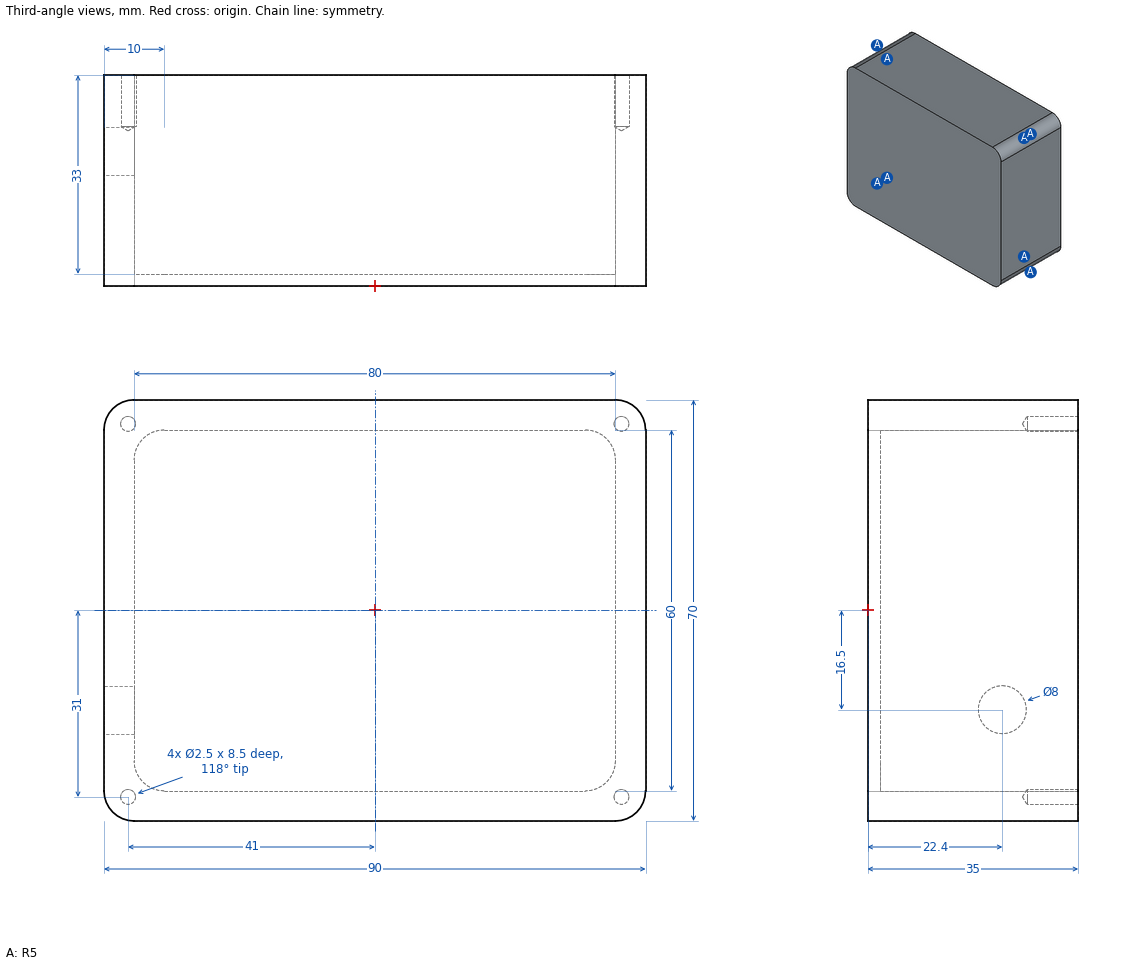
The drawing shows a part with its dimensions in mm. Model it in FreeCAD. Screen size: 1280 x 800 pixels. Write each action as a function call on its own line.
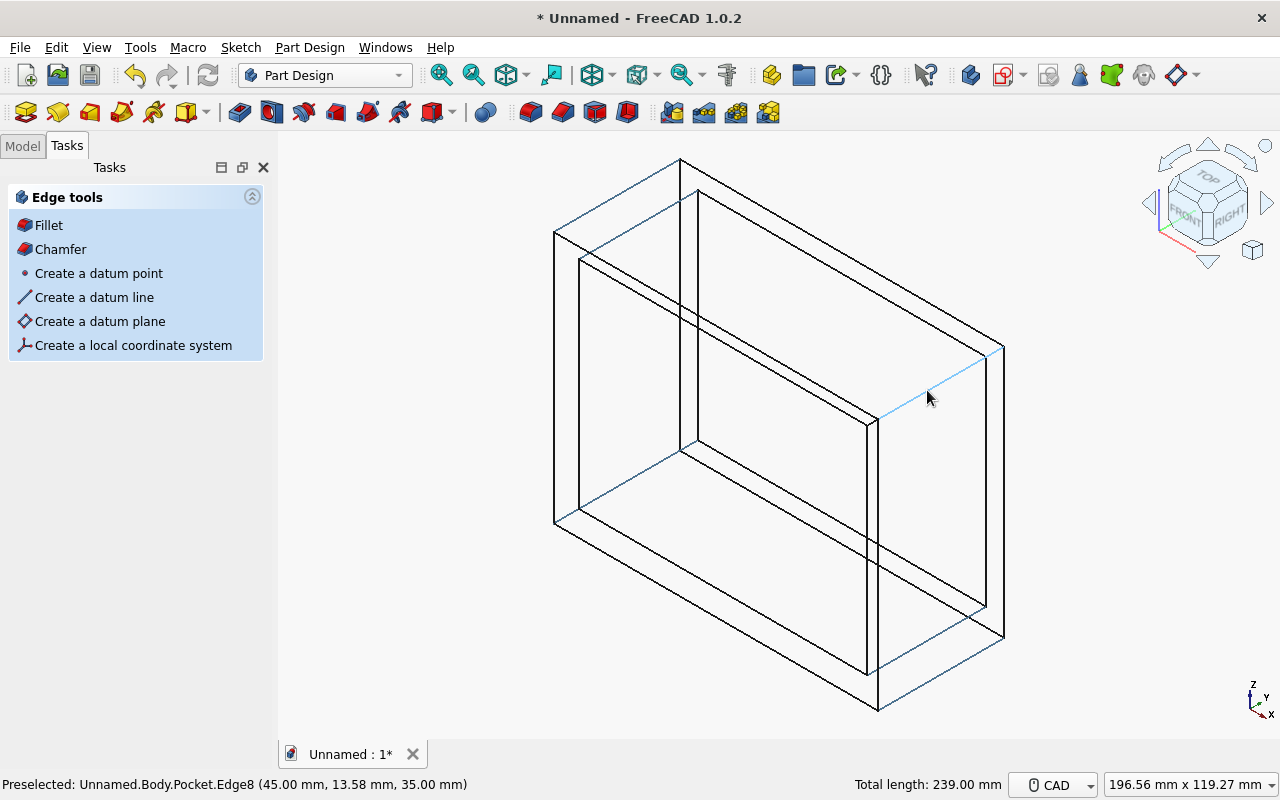
key(2)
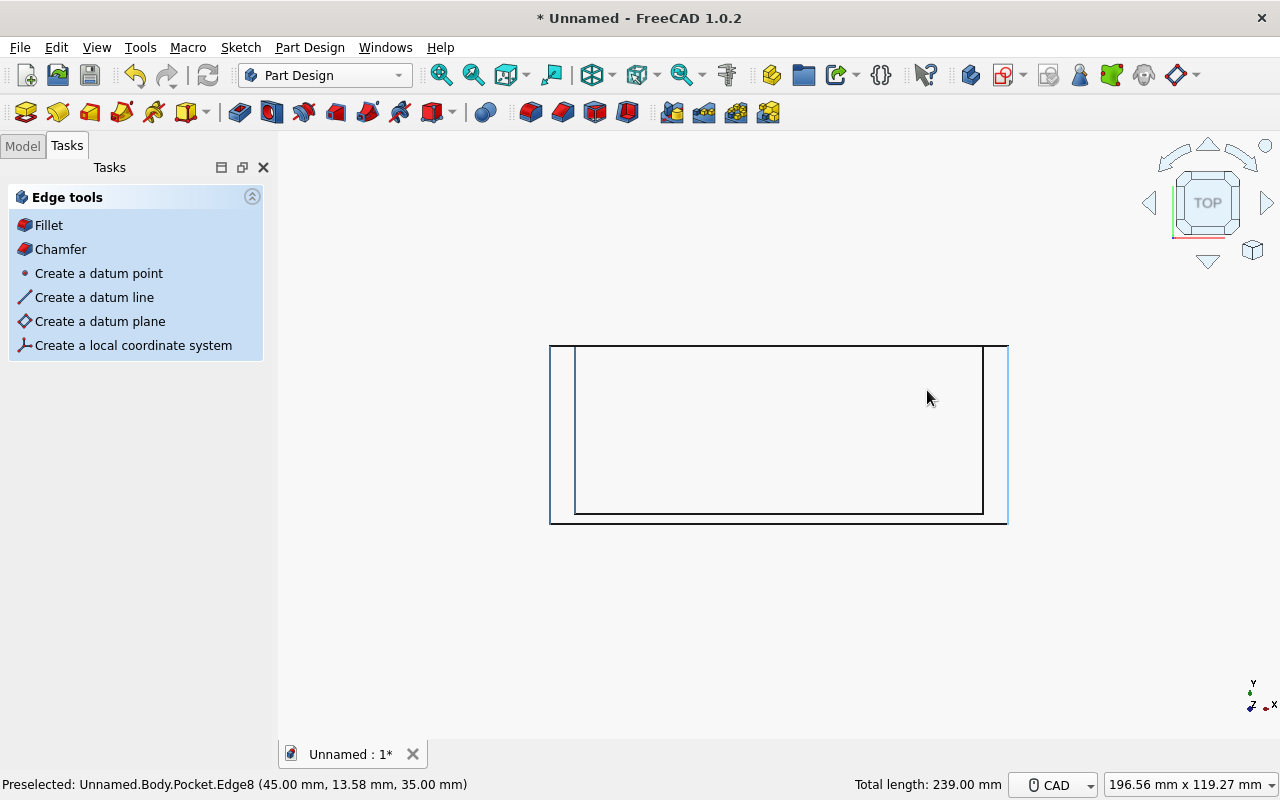
click(983, 429, ctrl)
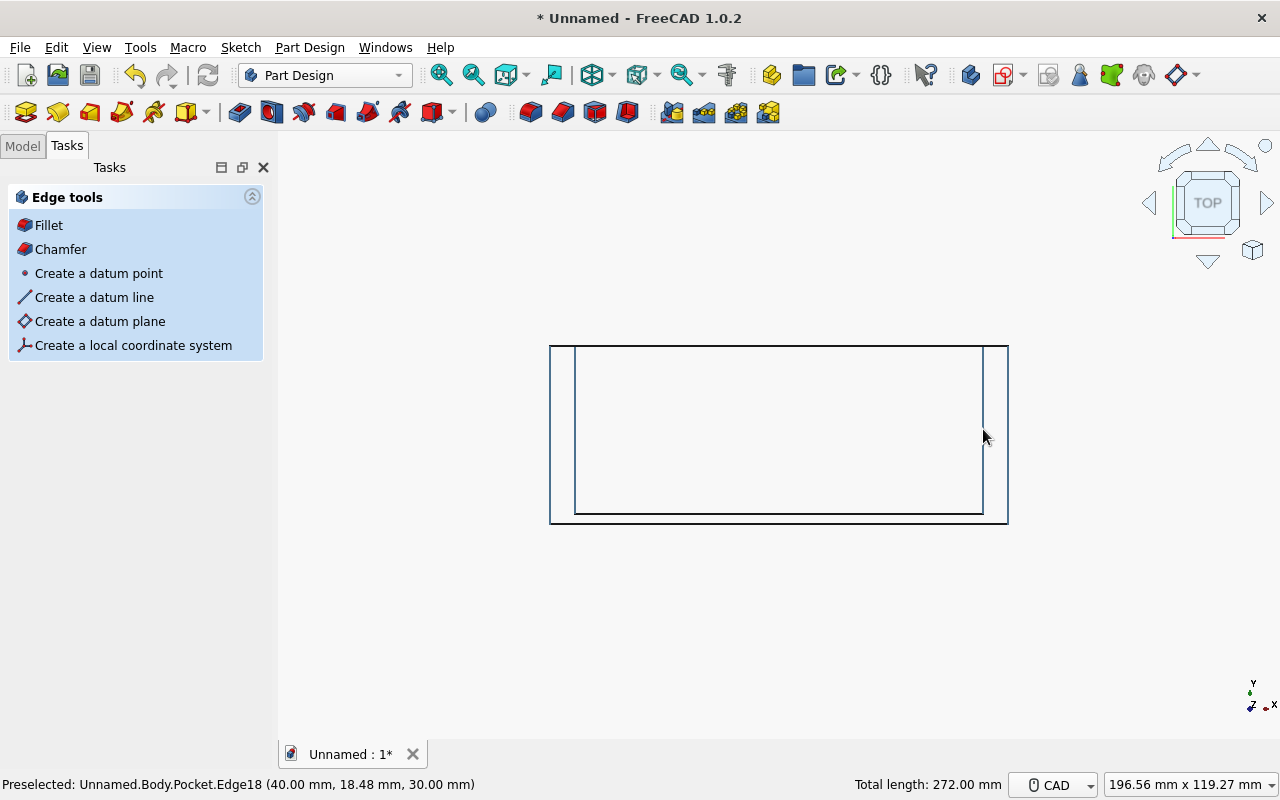
key(v)
key(1)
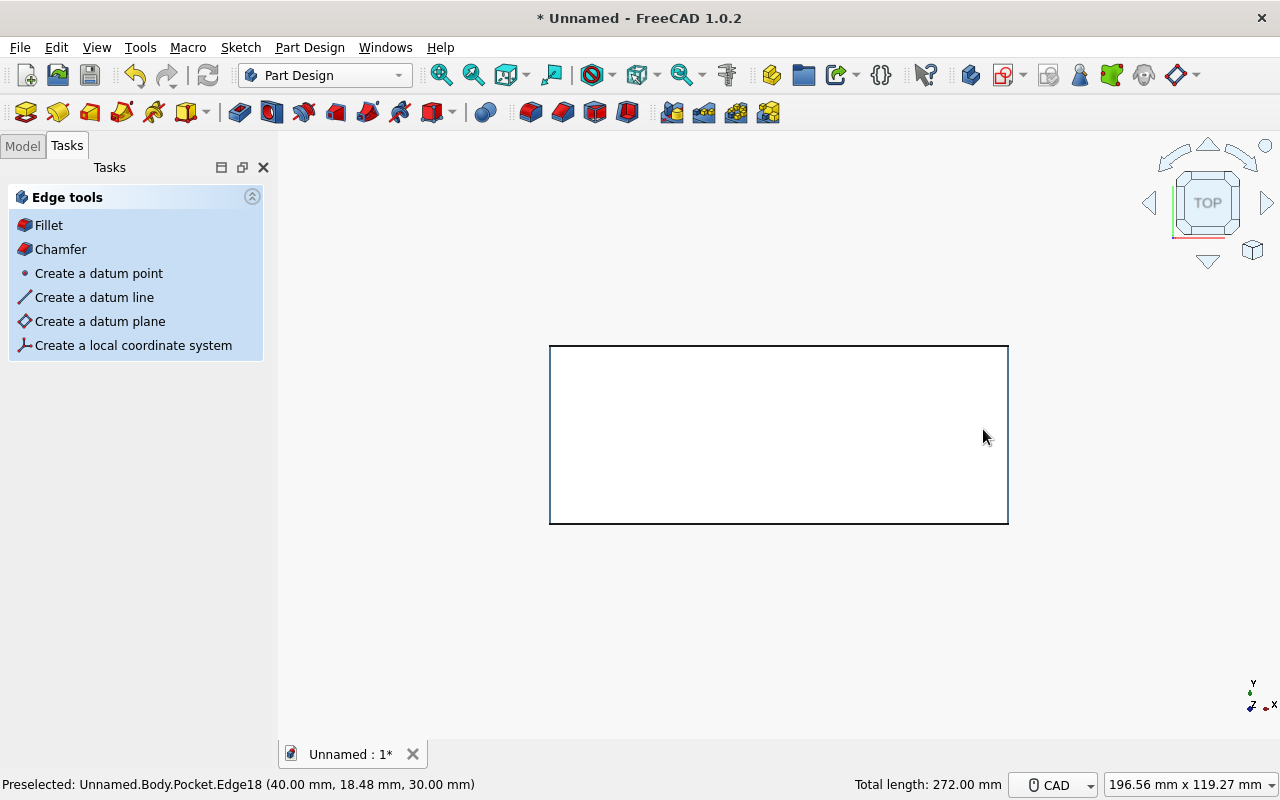
click(532, 112)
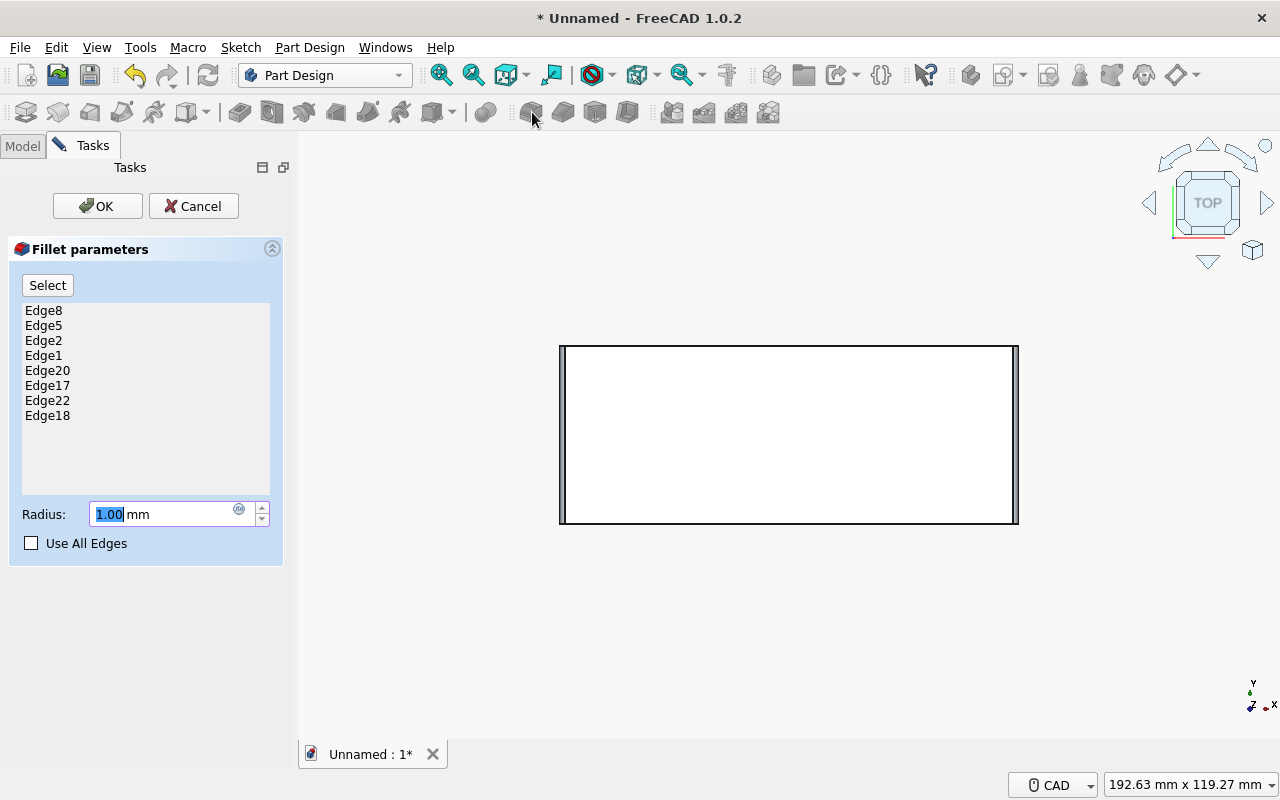
text(5)
key(Tab)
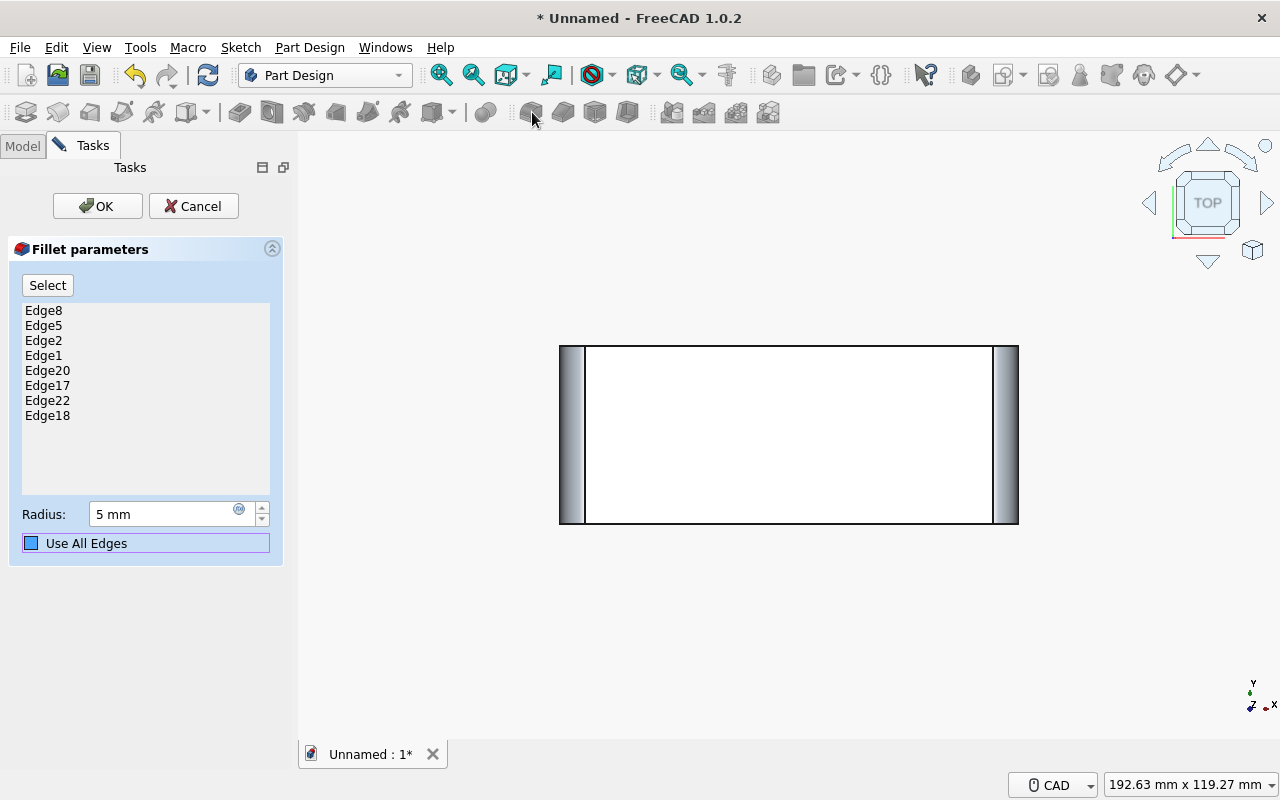
click(98, 206)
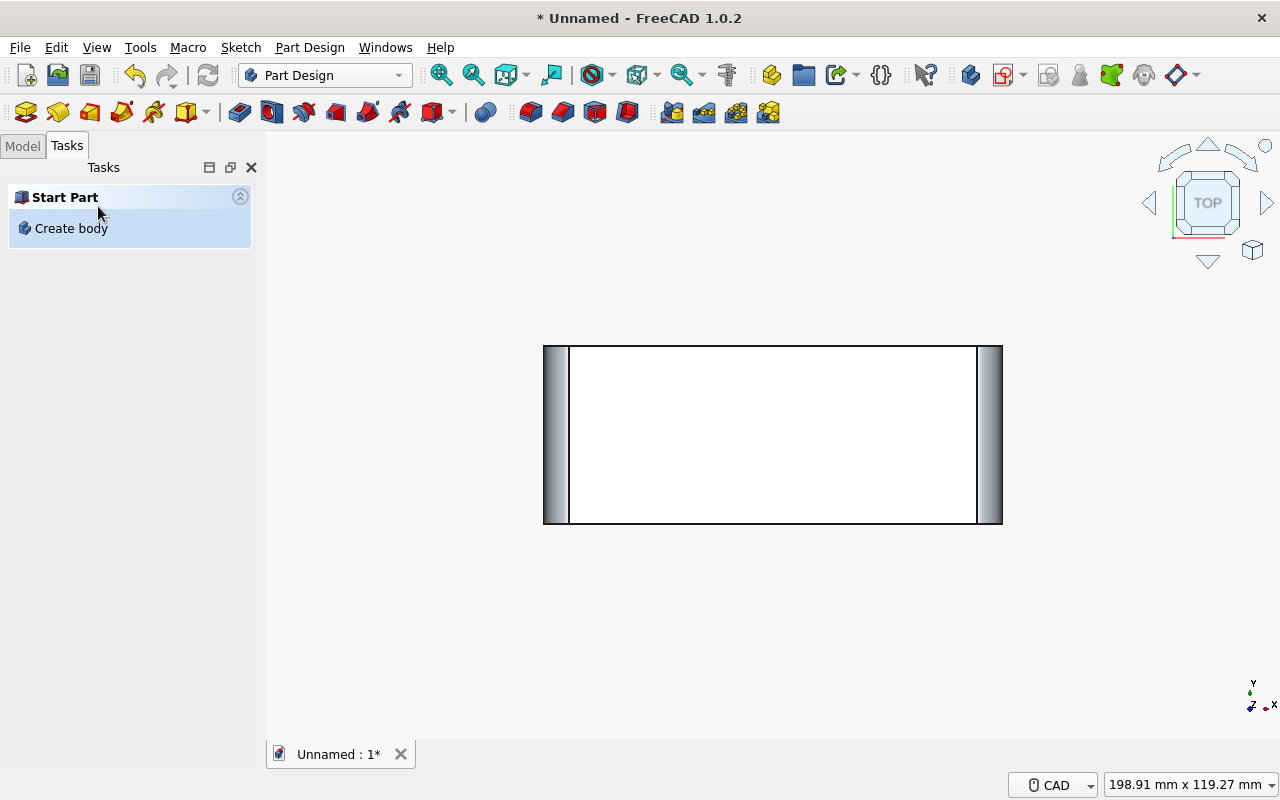
key(4)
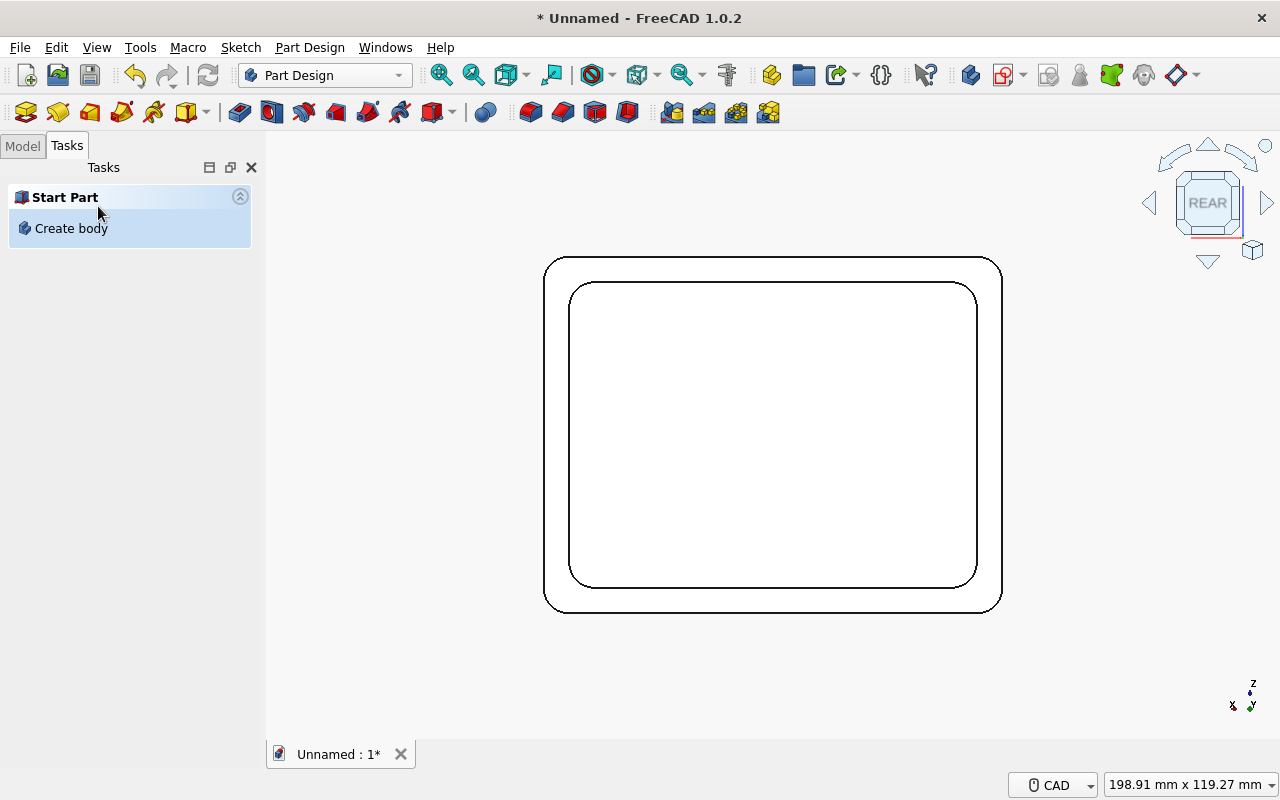
scroll(576, 587, up, 4)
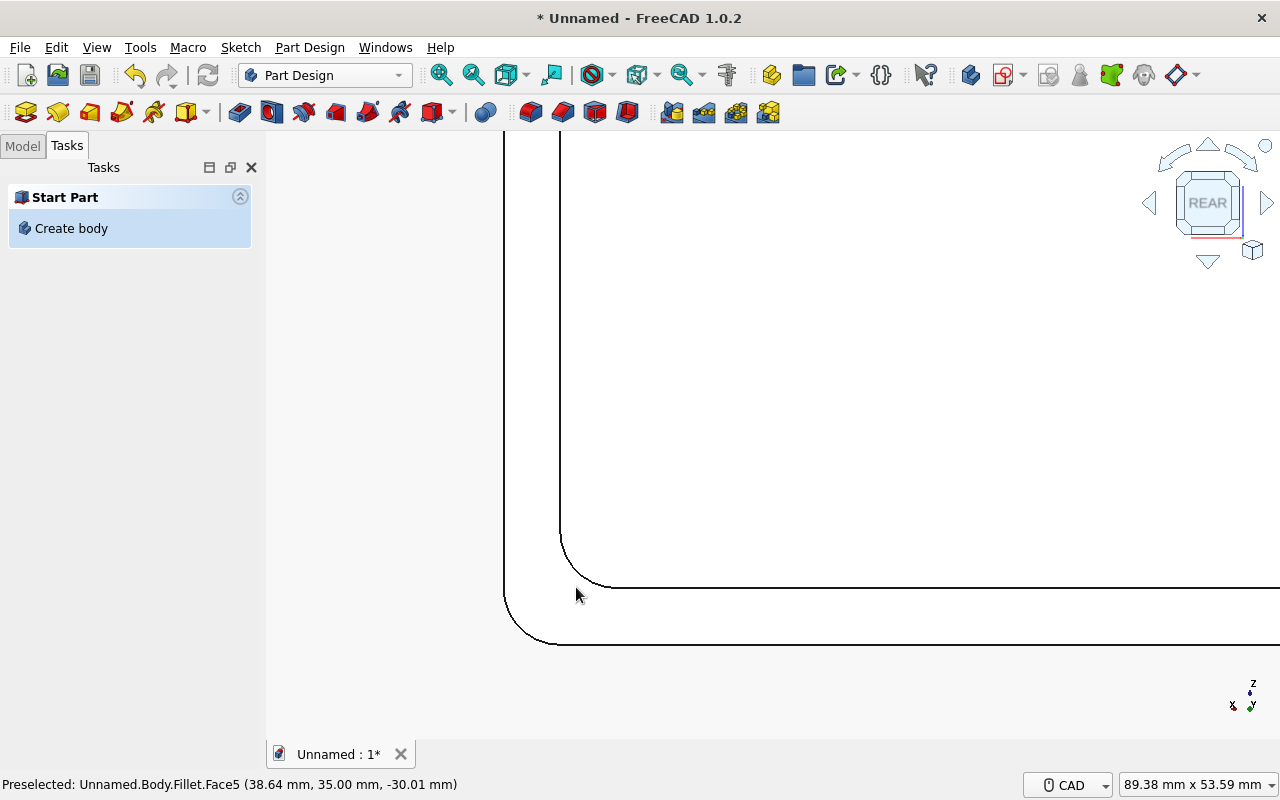
click(576, 587)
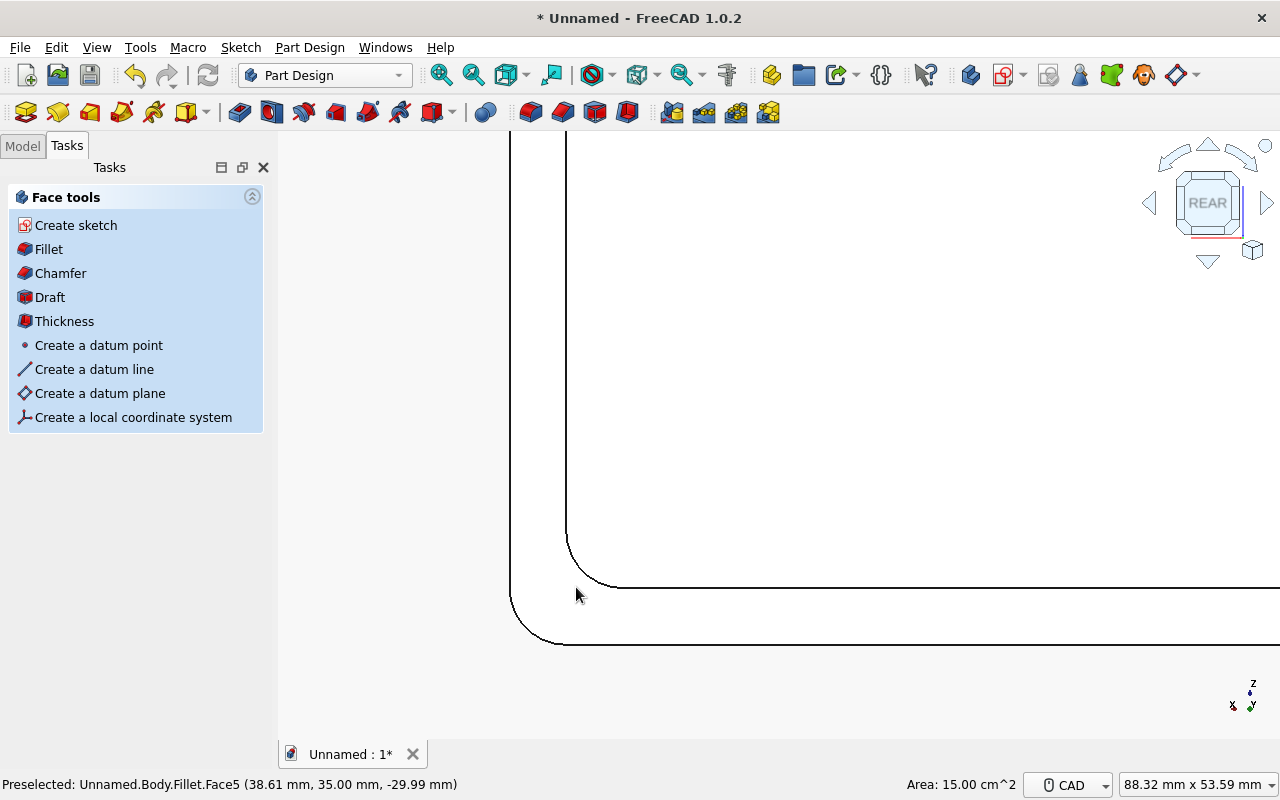
click(1004, 76)